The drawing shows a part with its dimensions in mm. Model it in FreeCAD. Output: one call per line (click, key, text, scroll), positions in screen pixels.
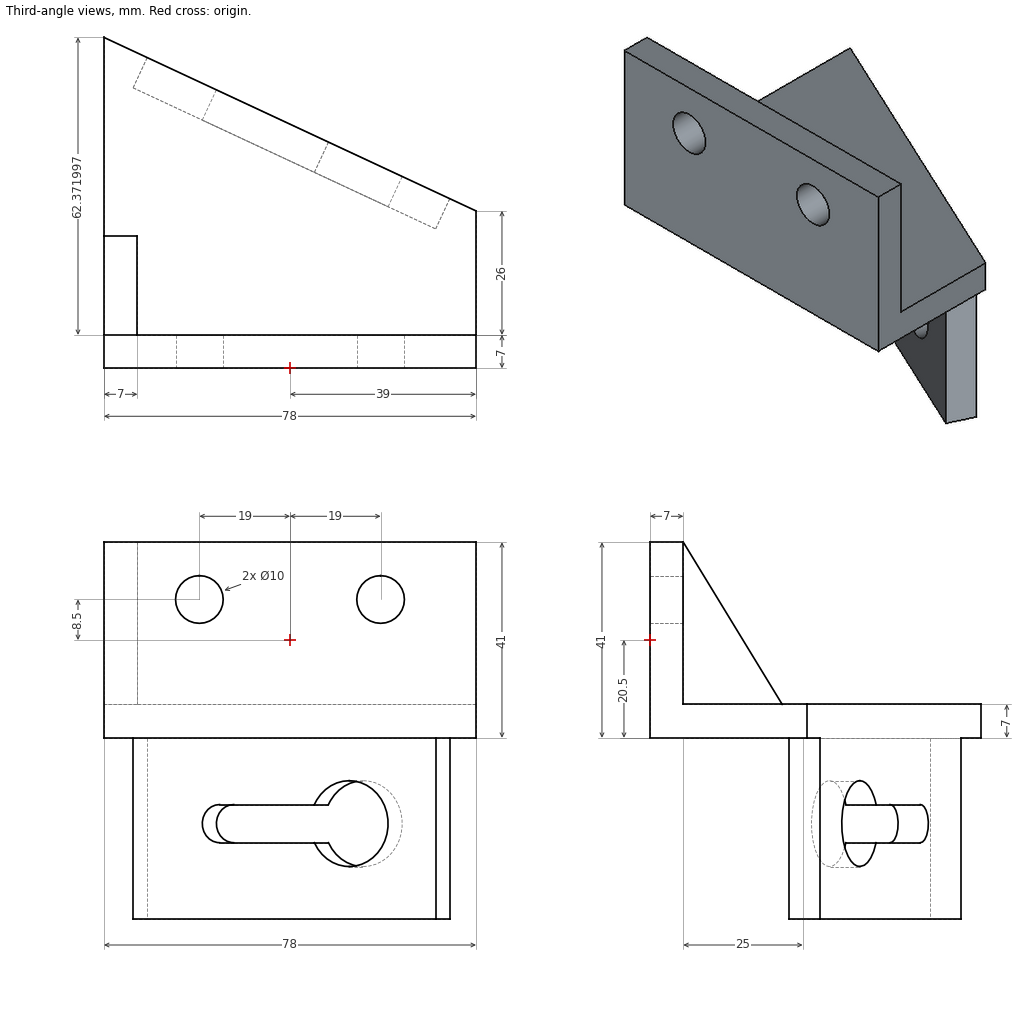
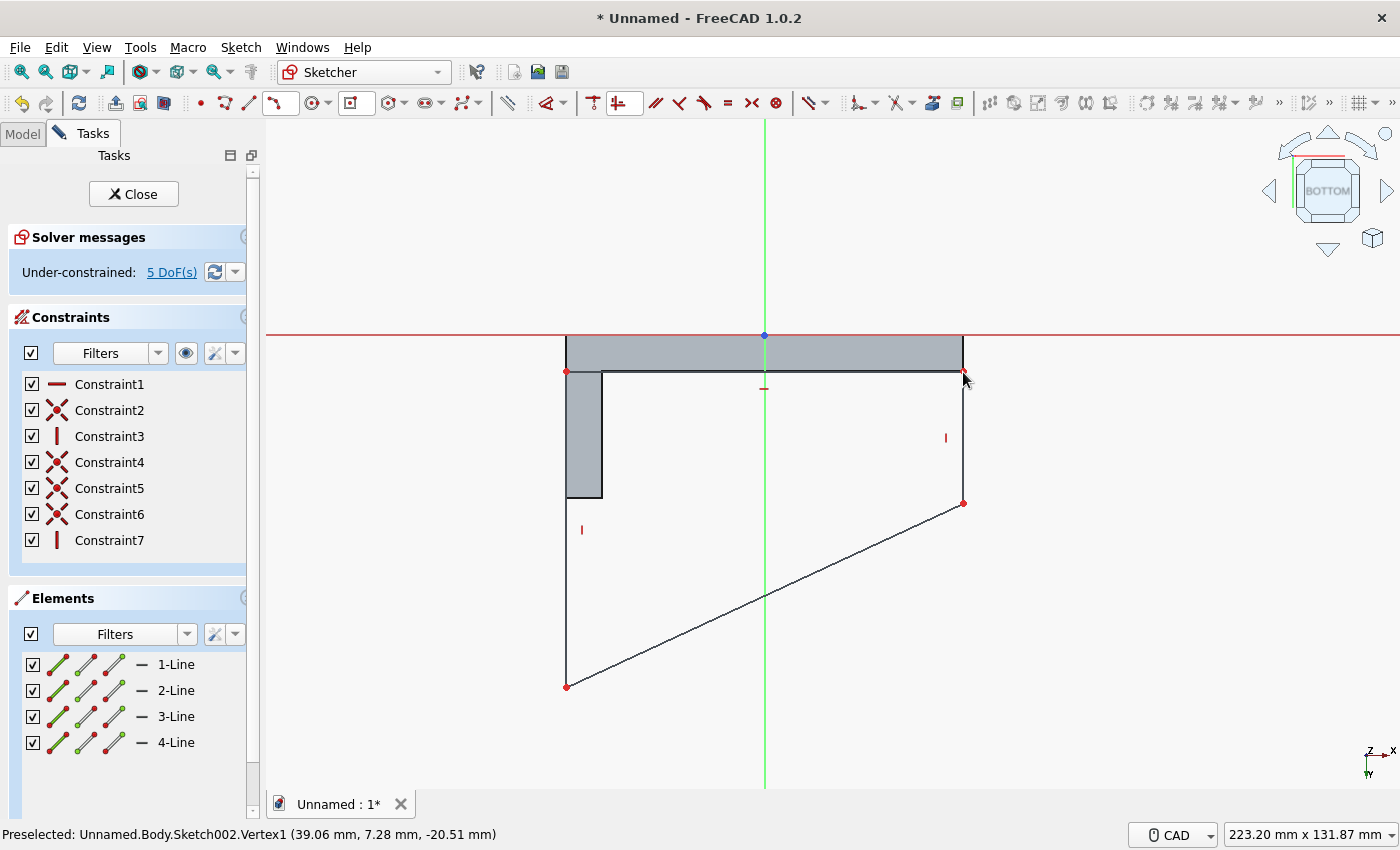
click(546, 104)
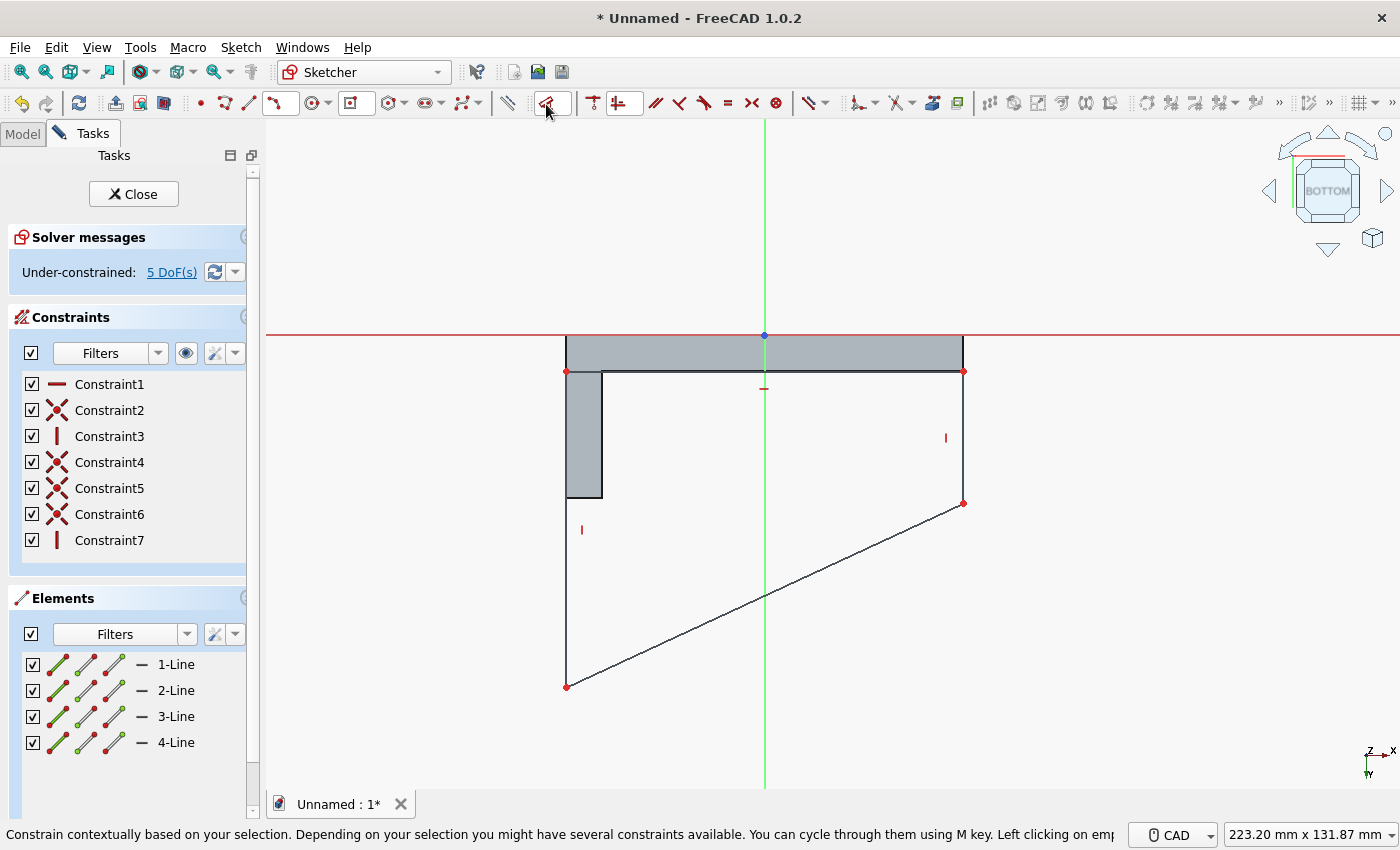
click(844, 372)
click(673, 406)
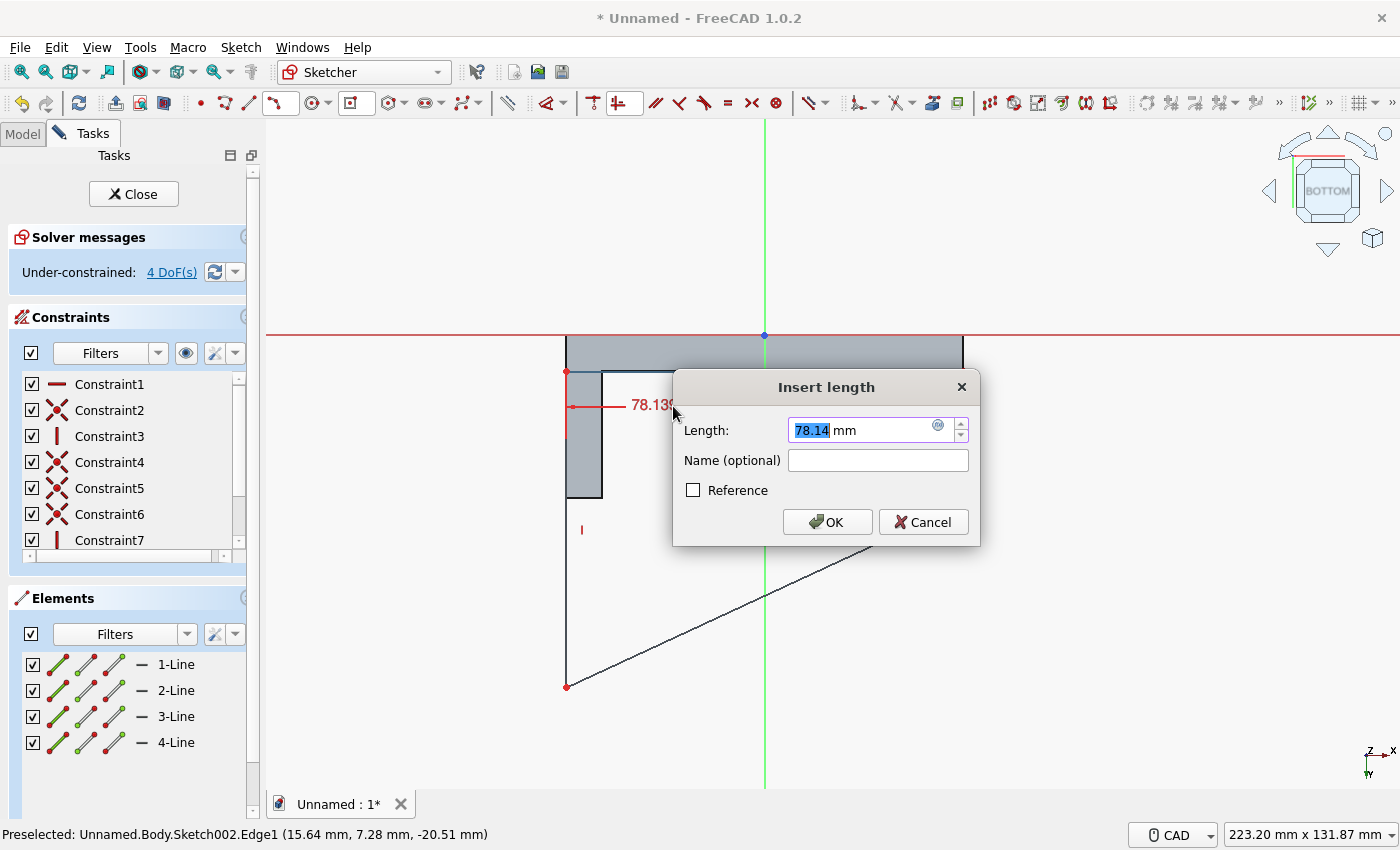
text(78)
key(Return)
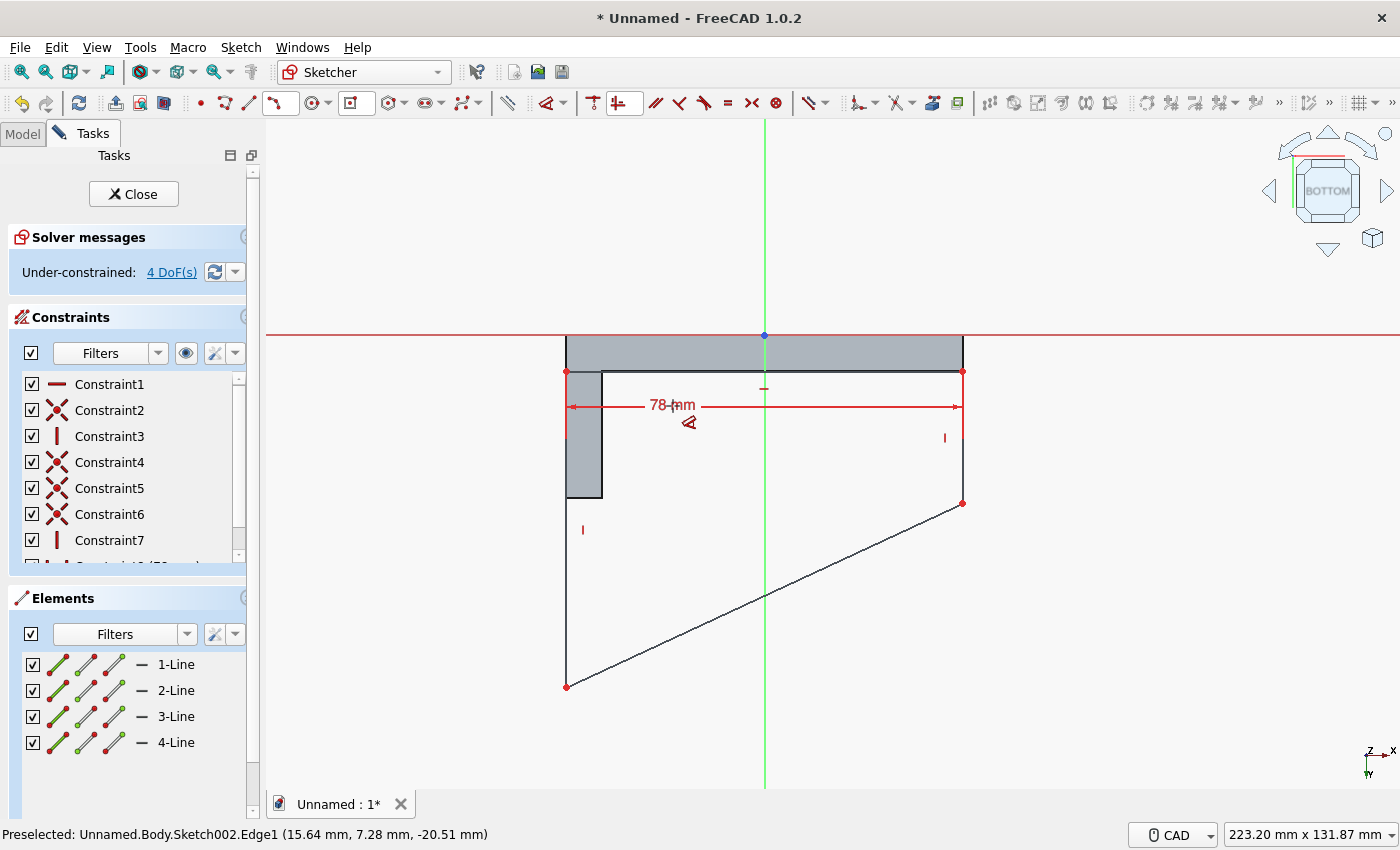
click(963, 464)
click(997, 438)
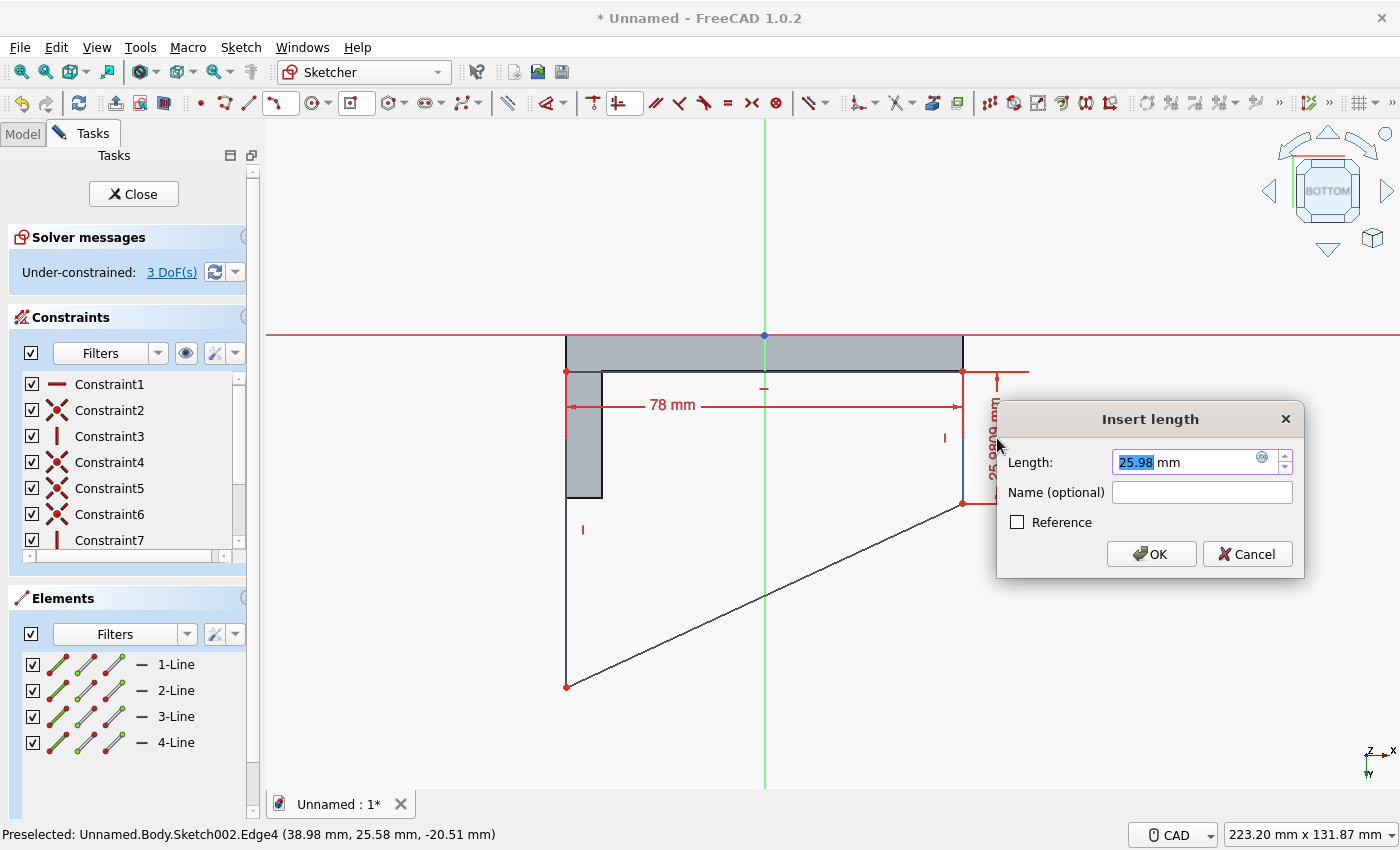
text(26)
key(Return)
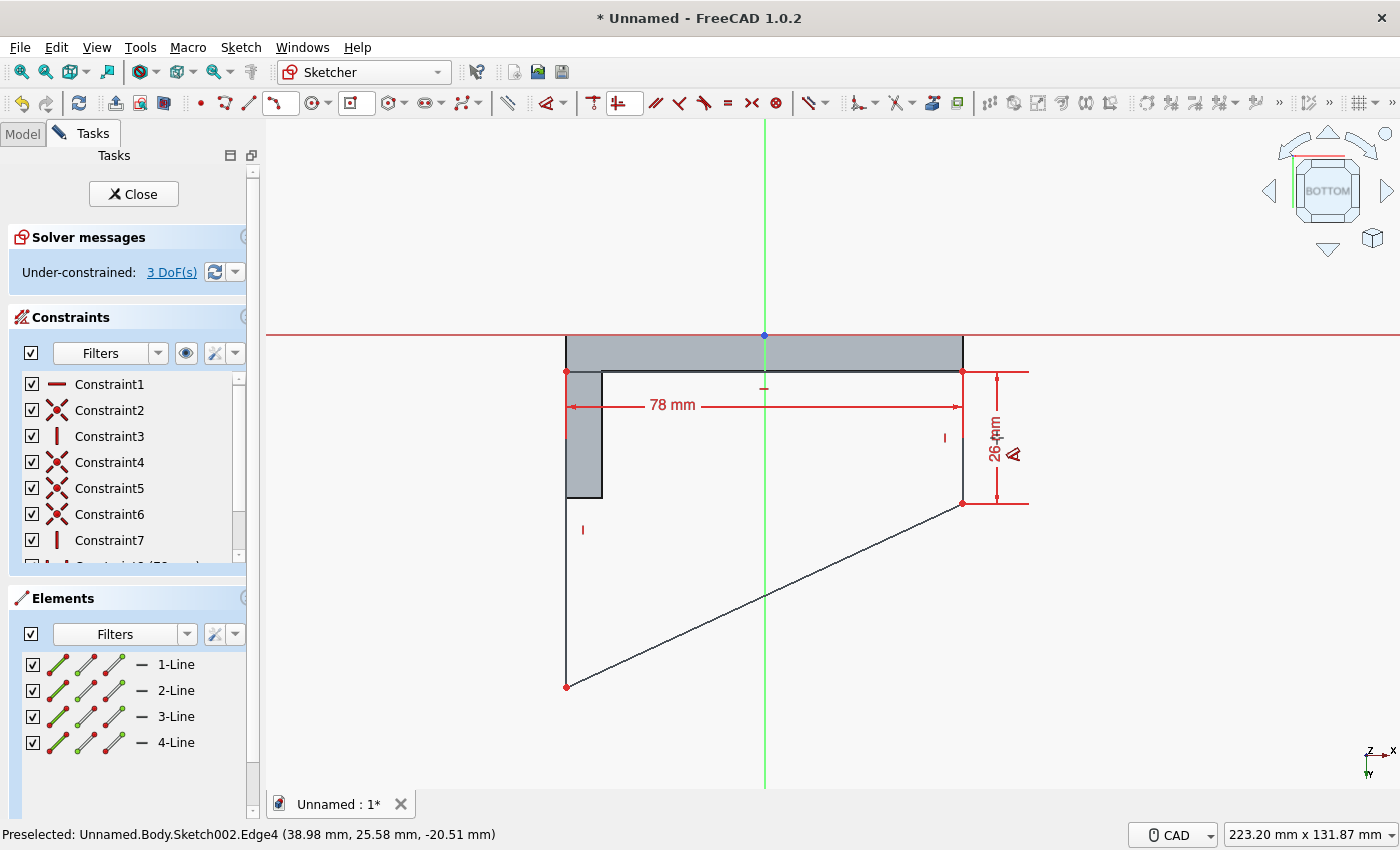
click(963, 372)
click(997, 353)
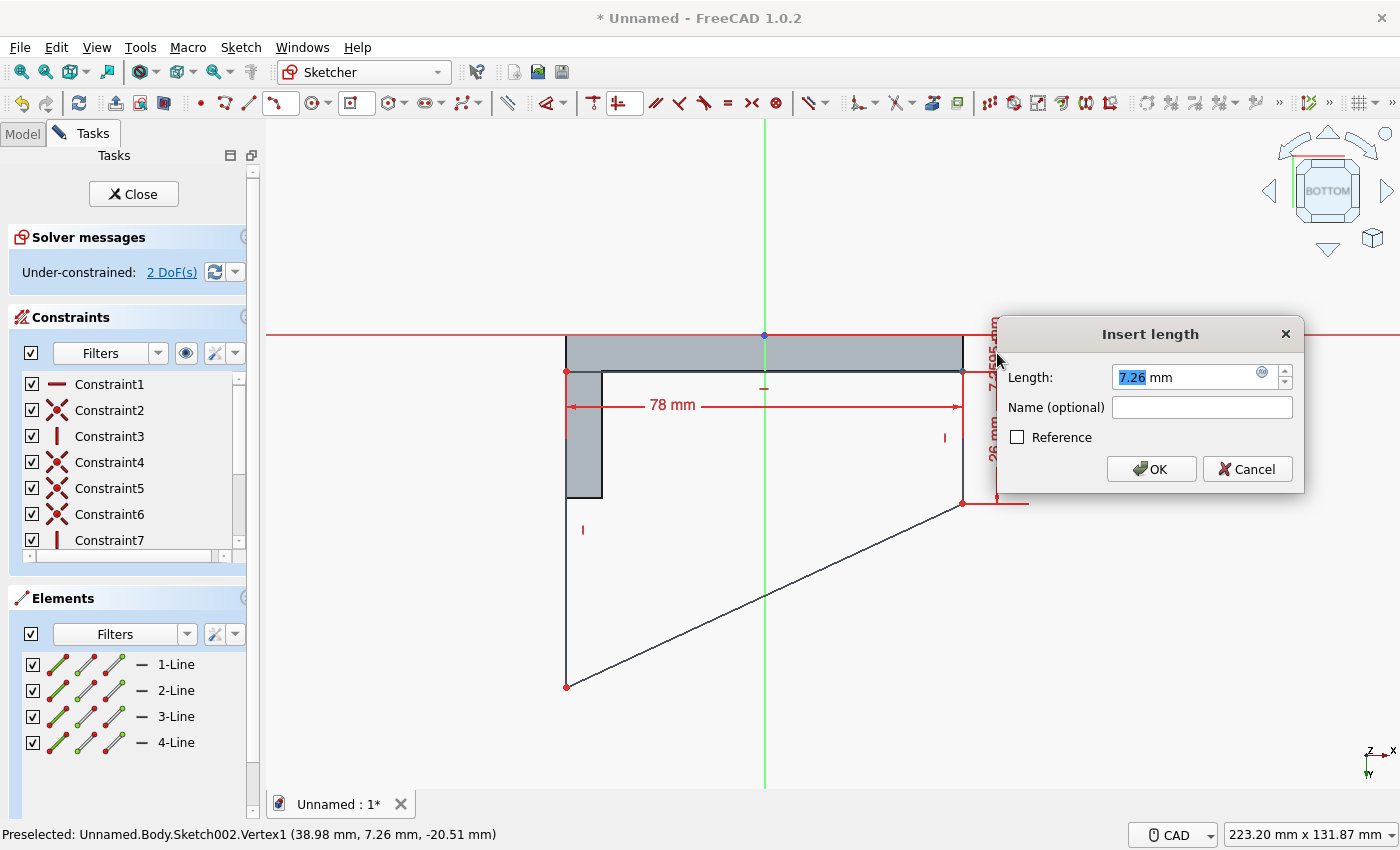
text(7)
key(Return)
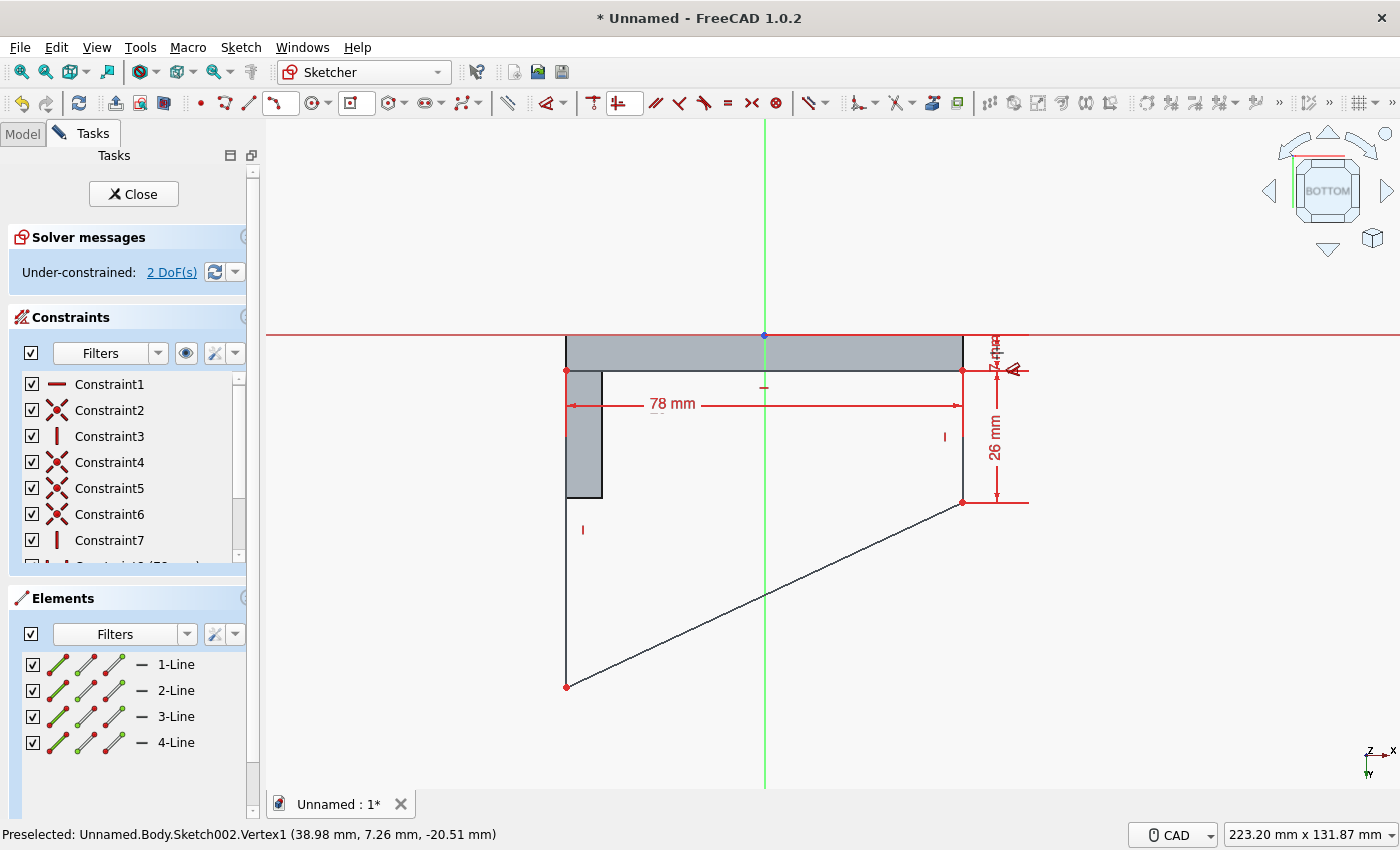
click(963, 371)
click(864, 301)